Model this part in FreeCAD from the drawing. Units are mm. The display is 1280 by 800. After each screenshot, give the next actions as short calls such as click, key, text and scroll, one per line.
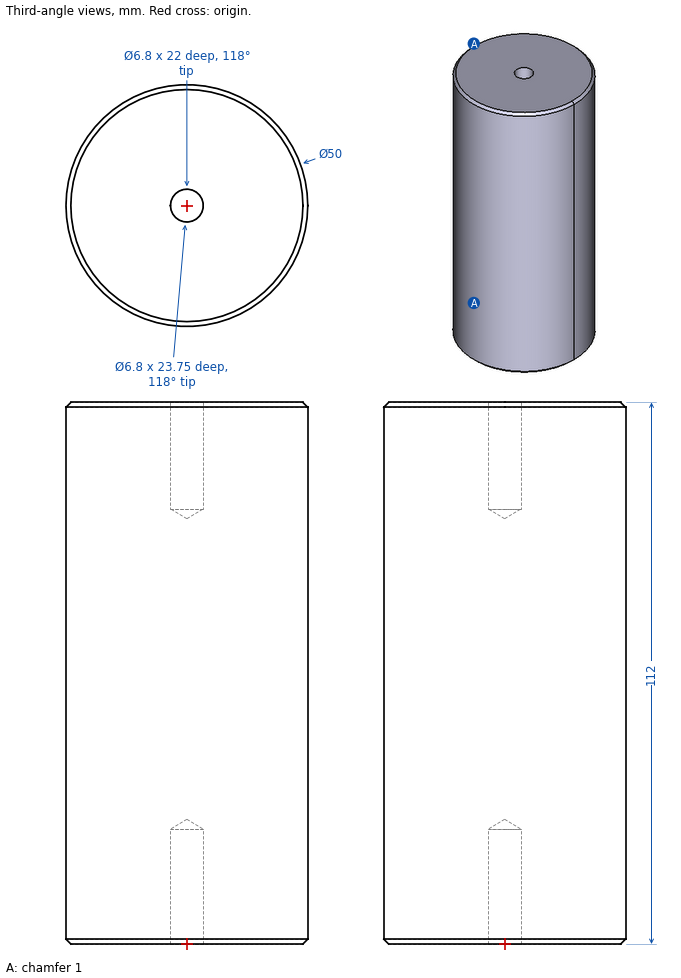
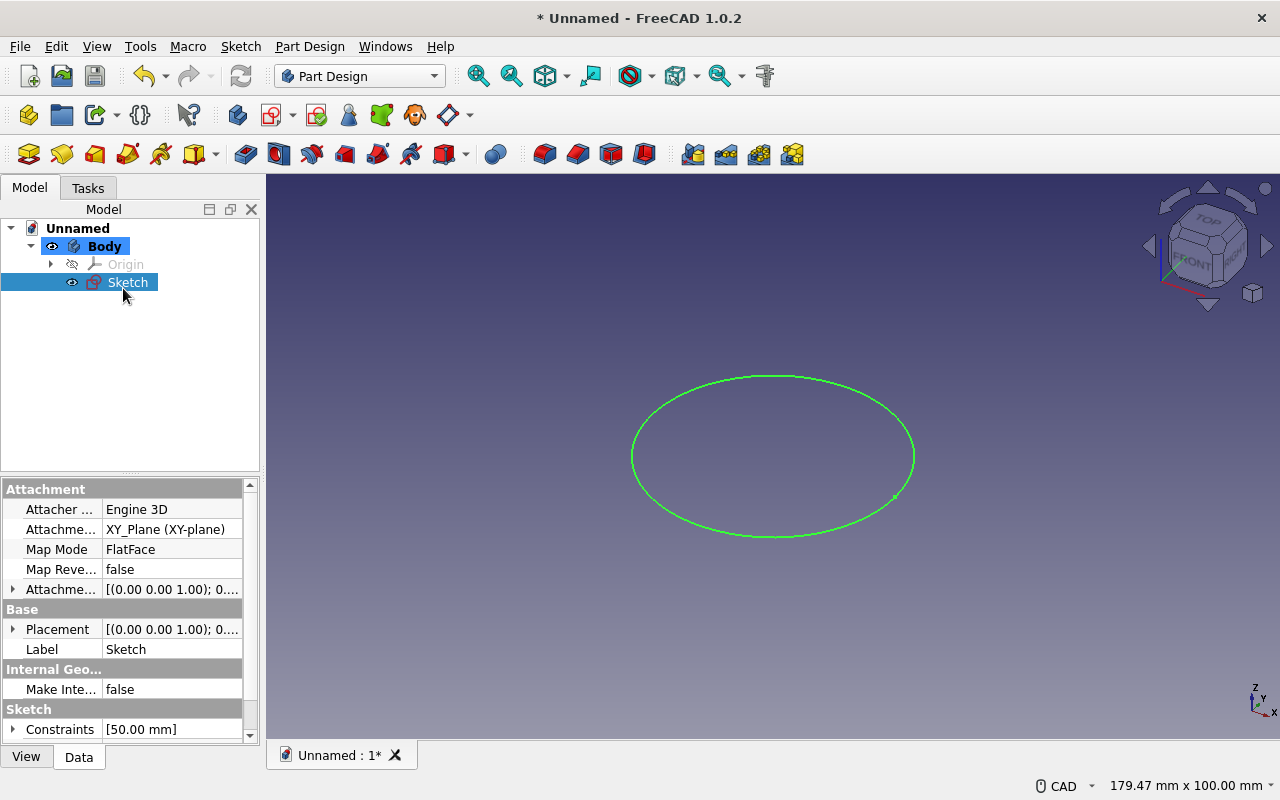
click(29, 154)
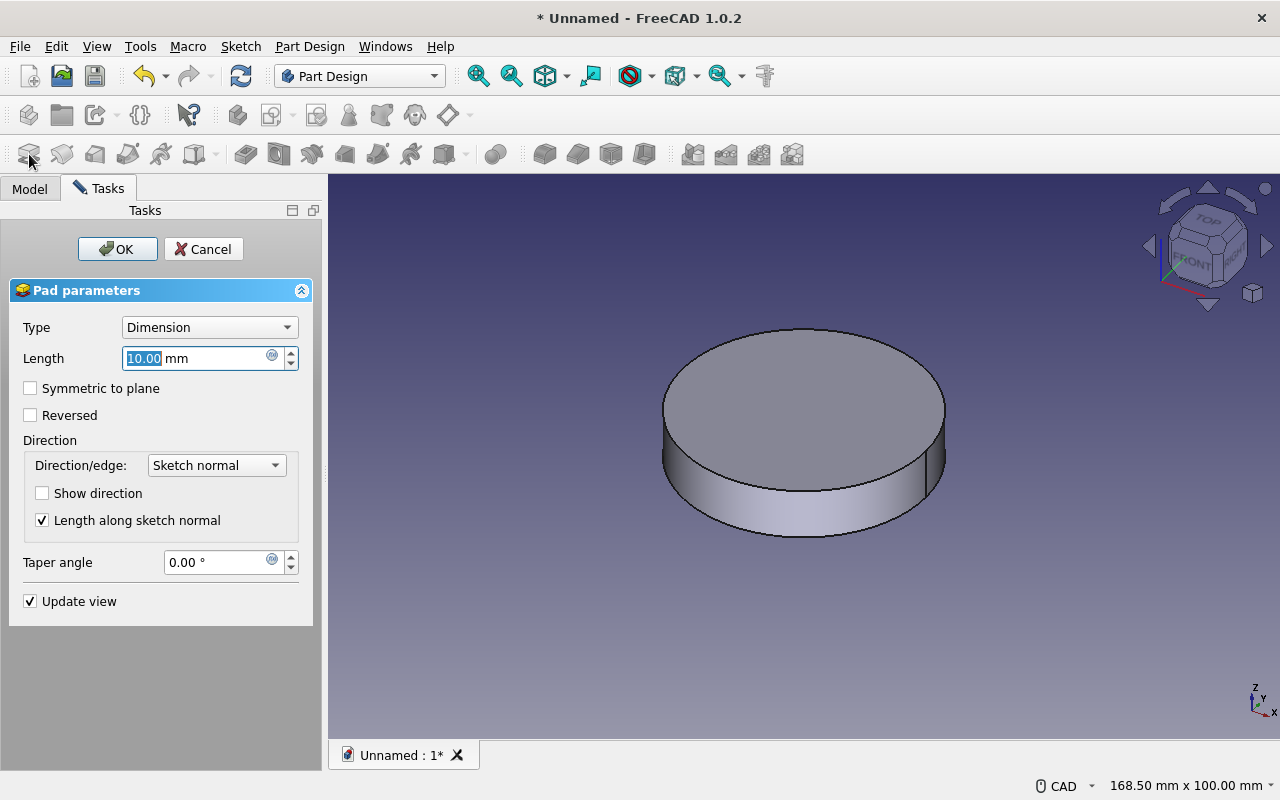
text(112)
key(Tab)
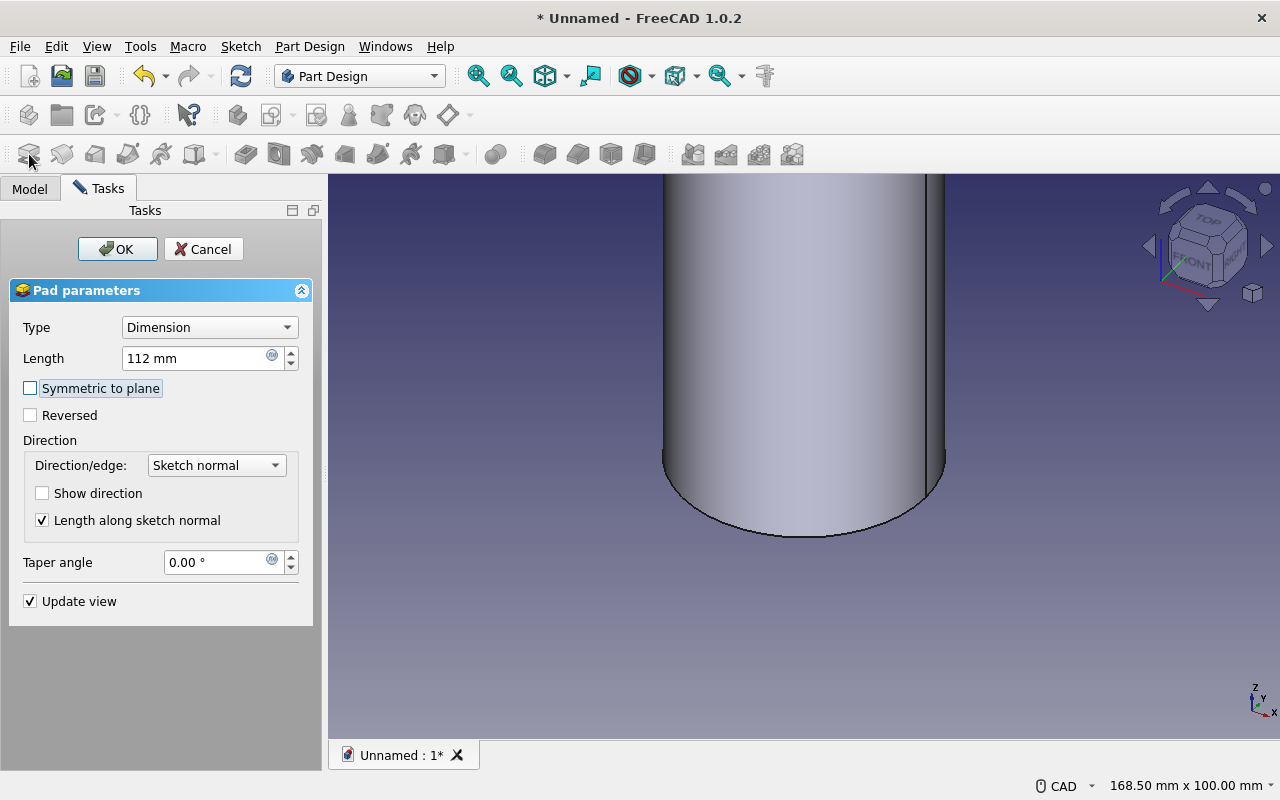
click(118, 249)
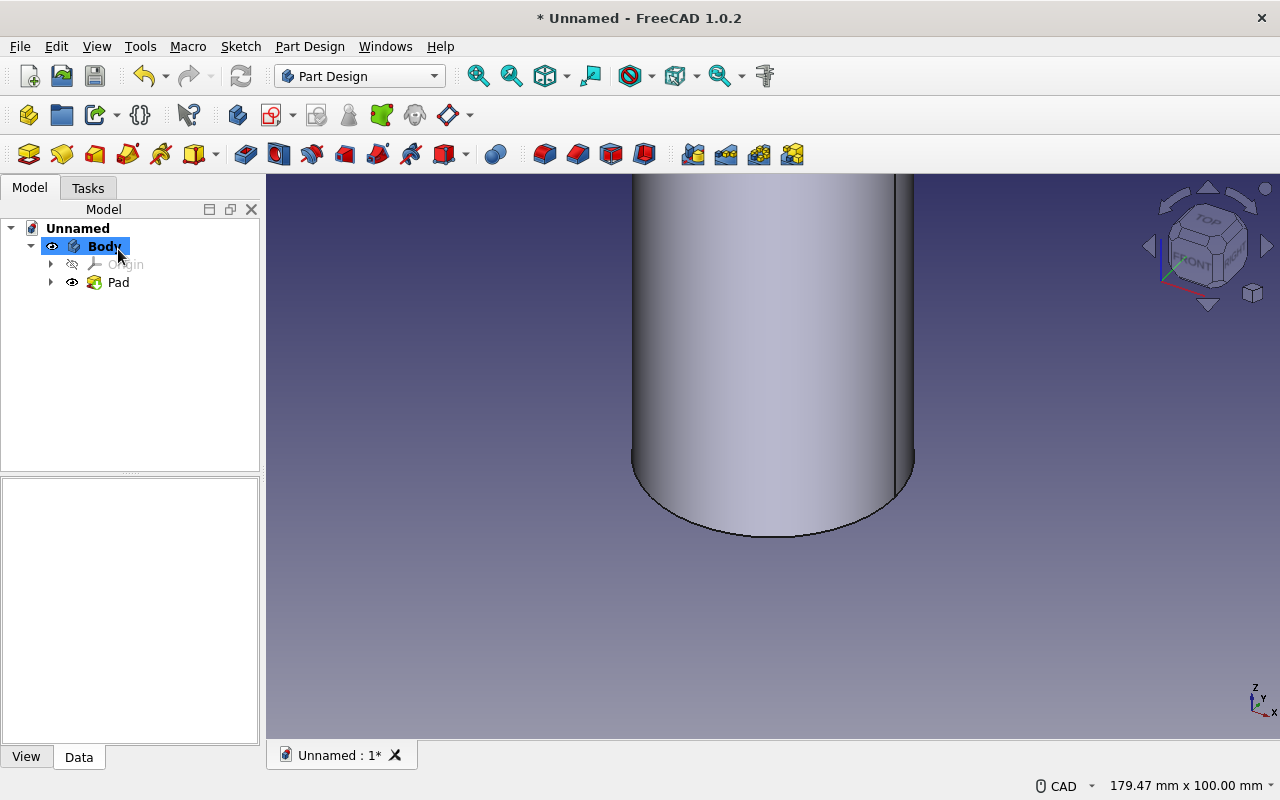
key(v)
key(f)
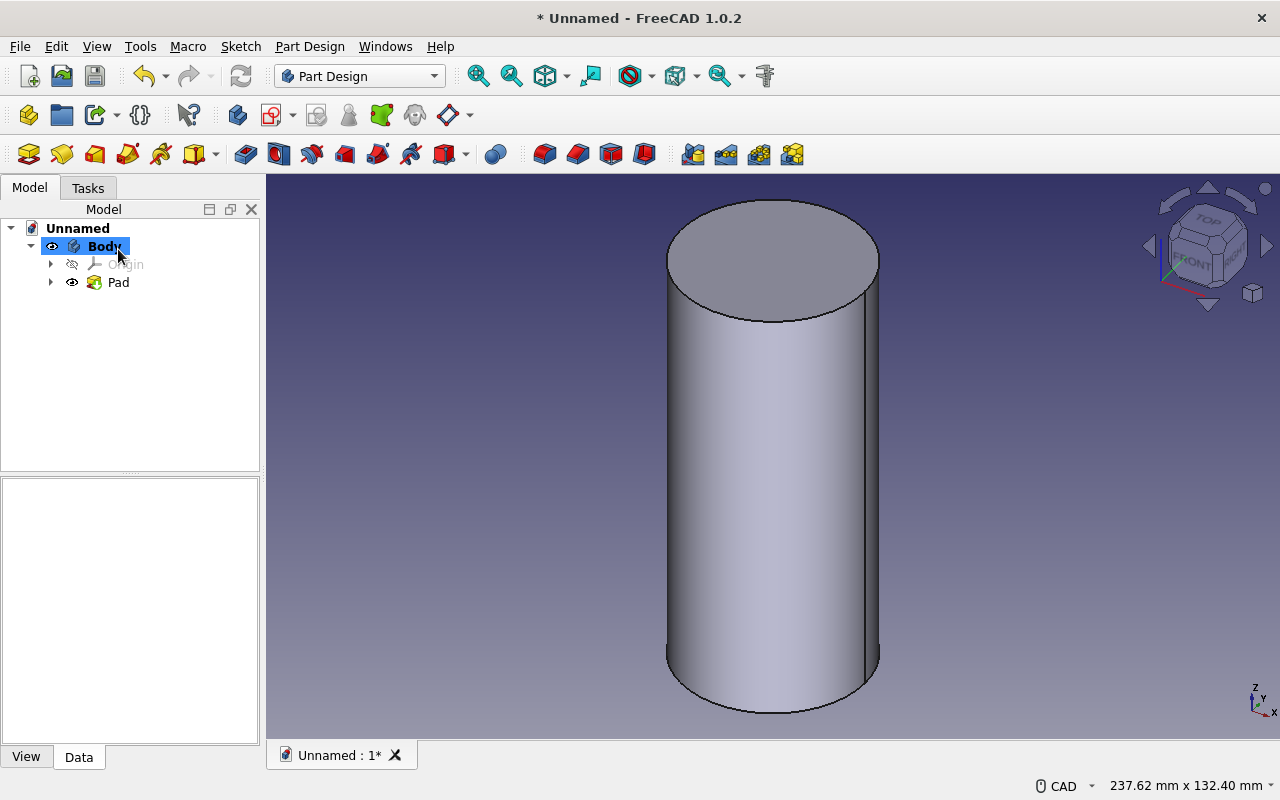
click(773, 260)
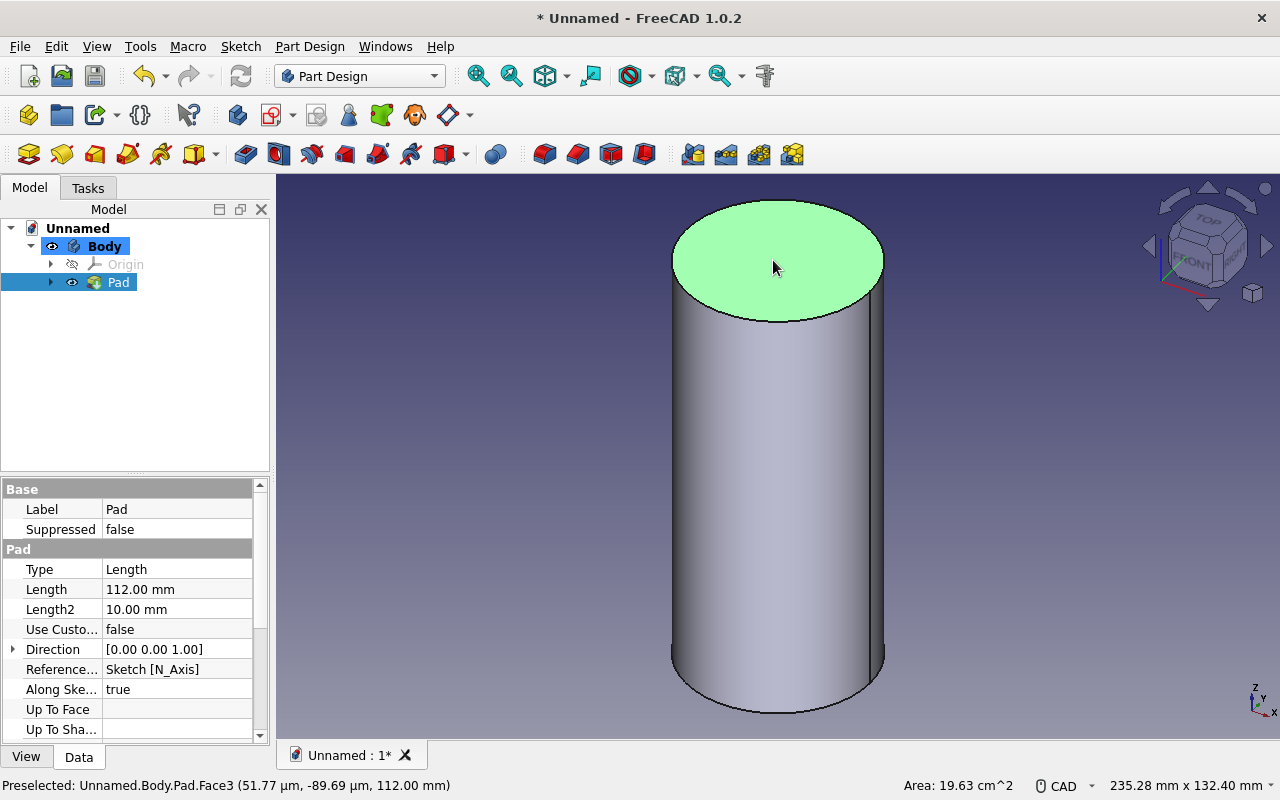
click(270, 116)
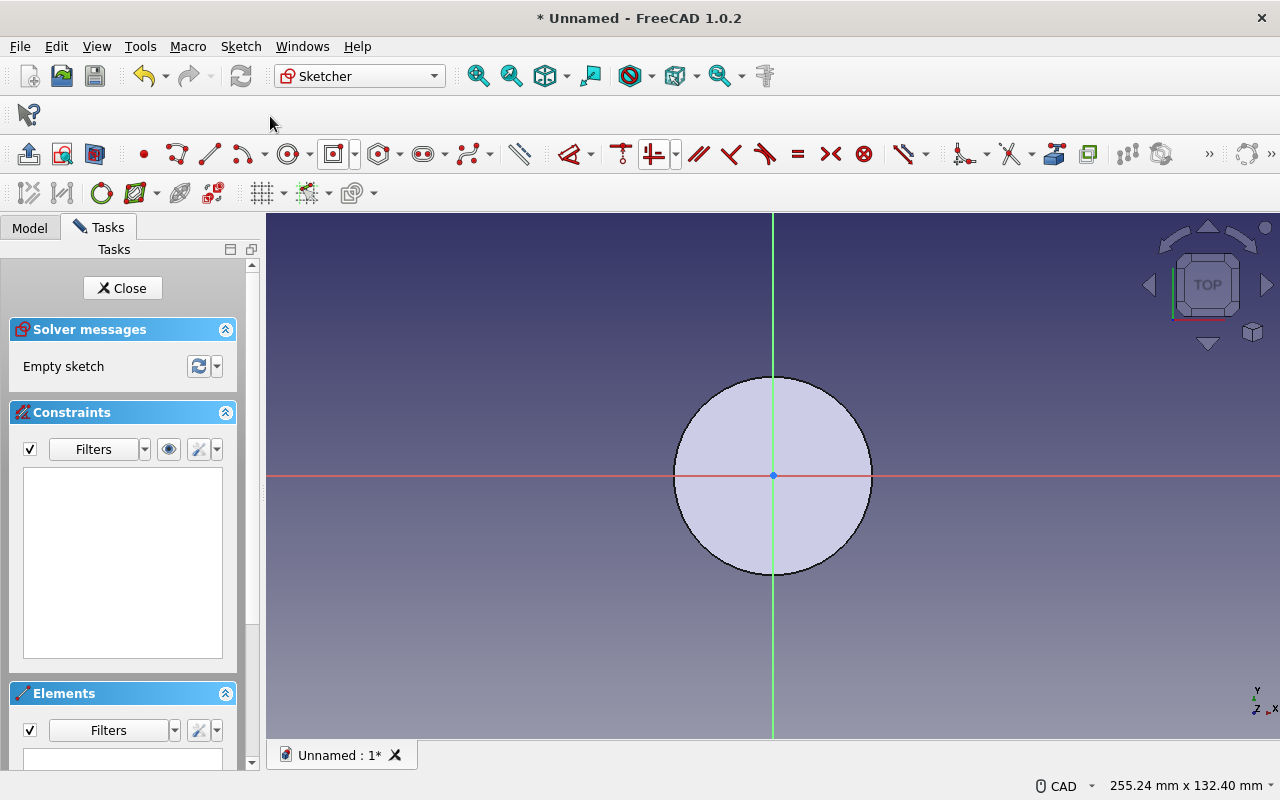
scroll(778, 476, up, 13)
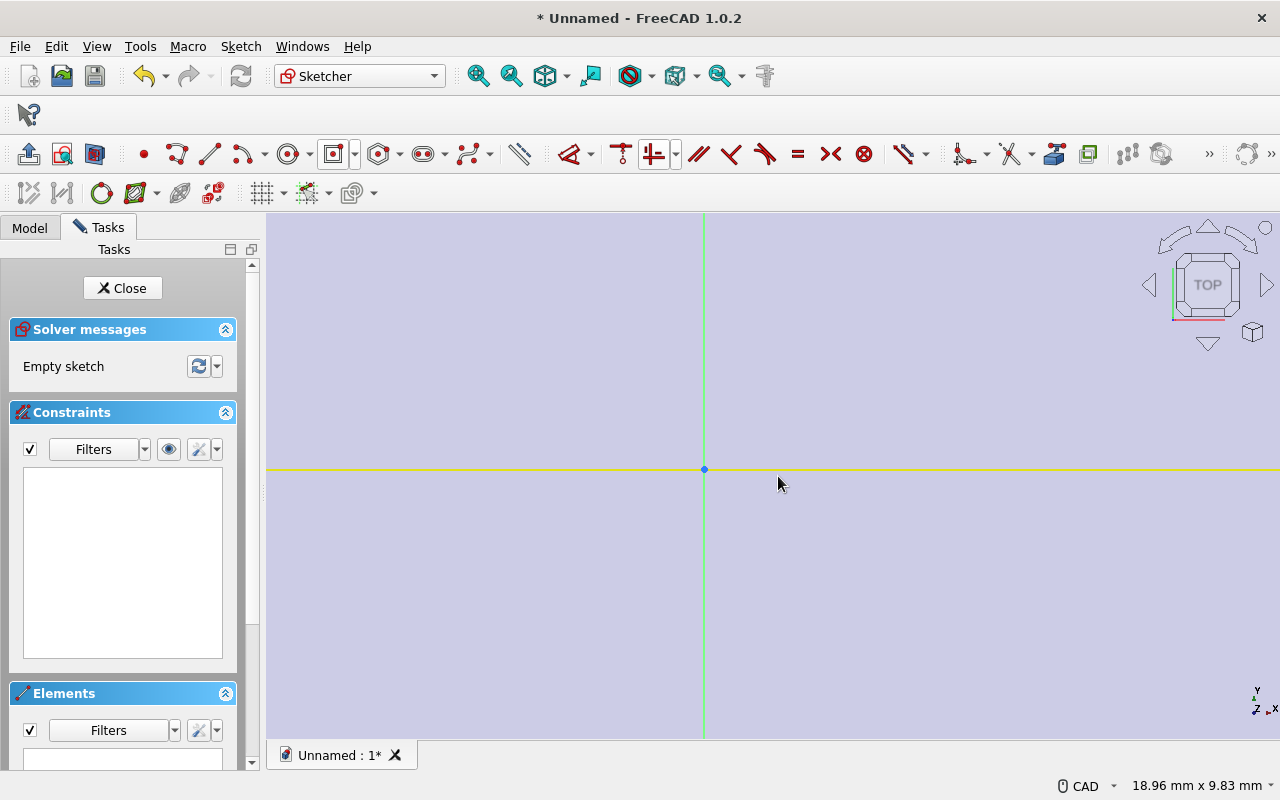
key(g)
key(c)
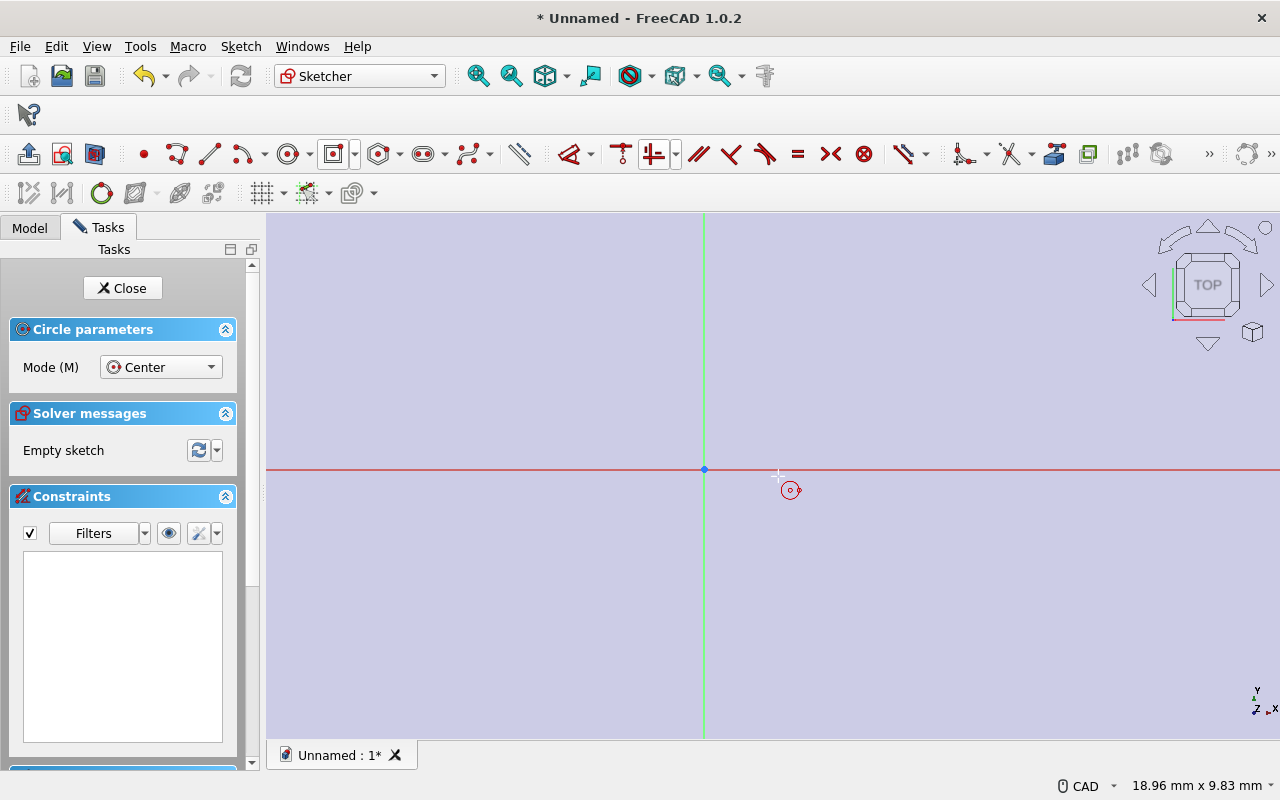
click(704, 470)
click(833, 341)
key(Escape)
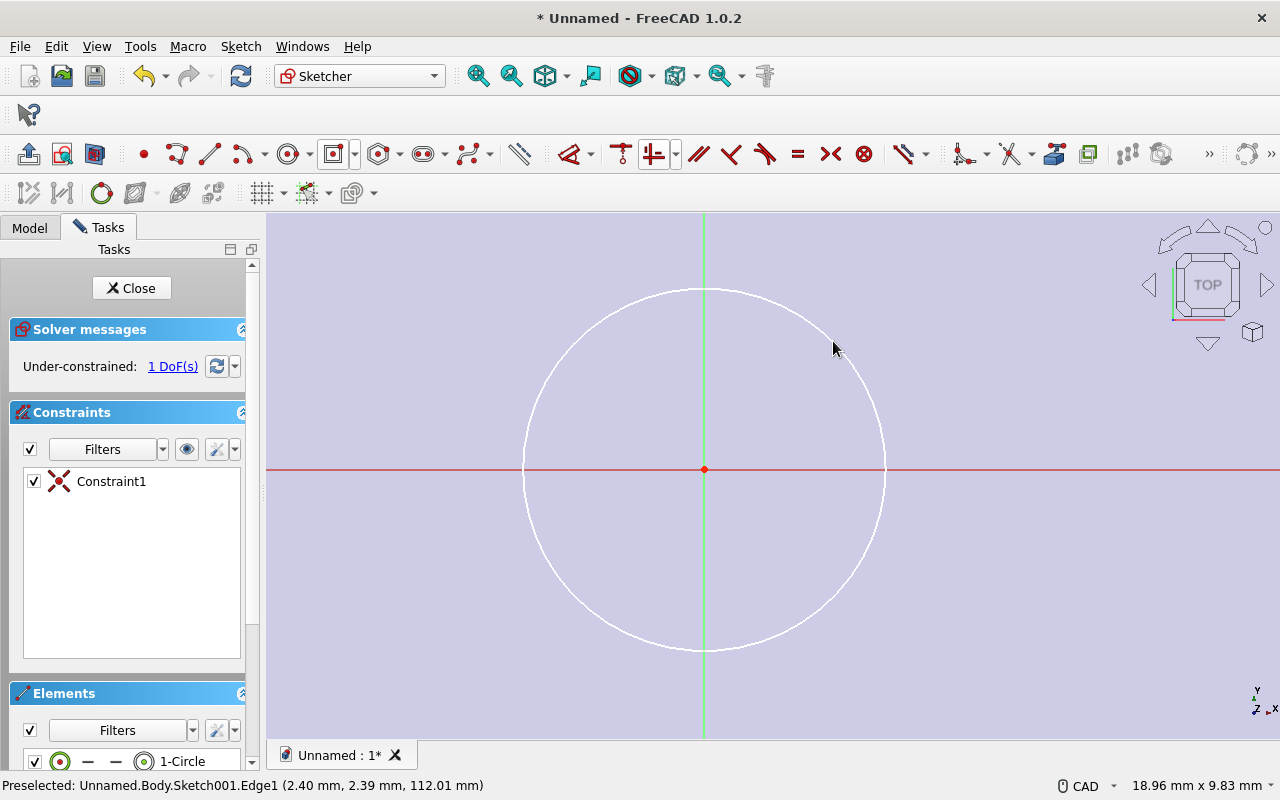
click(568, 154)